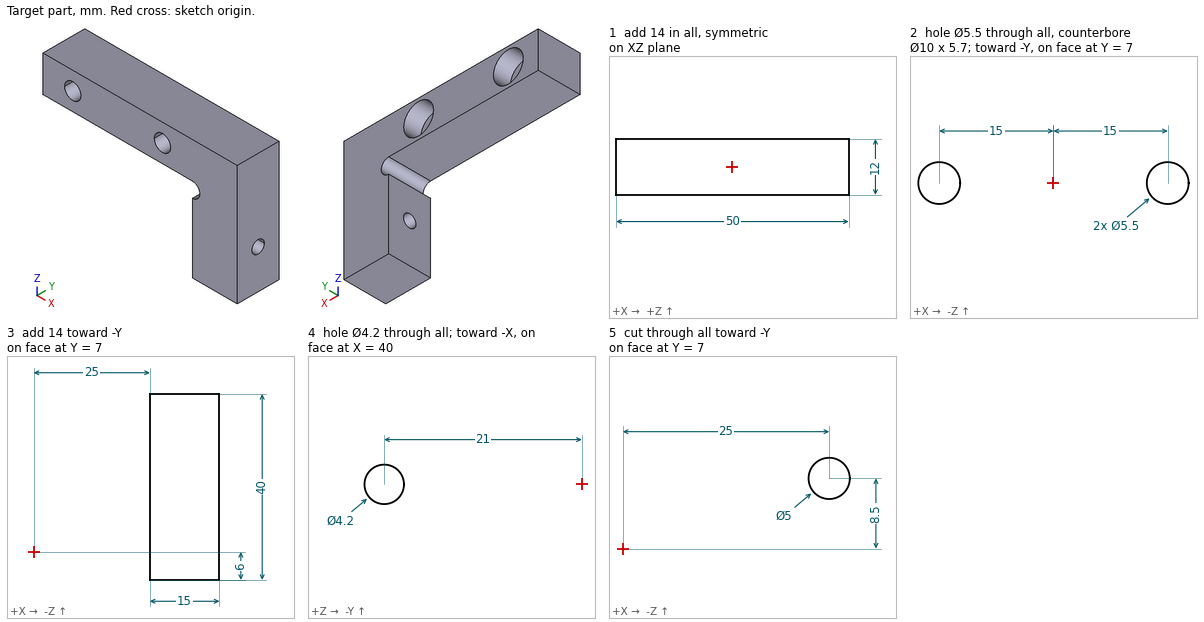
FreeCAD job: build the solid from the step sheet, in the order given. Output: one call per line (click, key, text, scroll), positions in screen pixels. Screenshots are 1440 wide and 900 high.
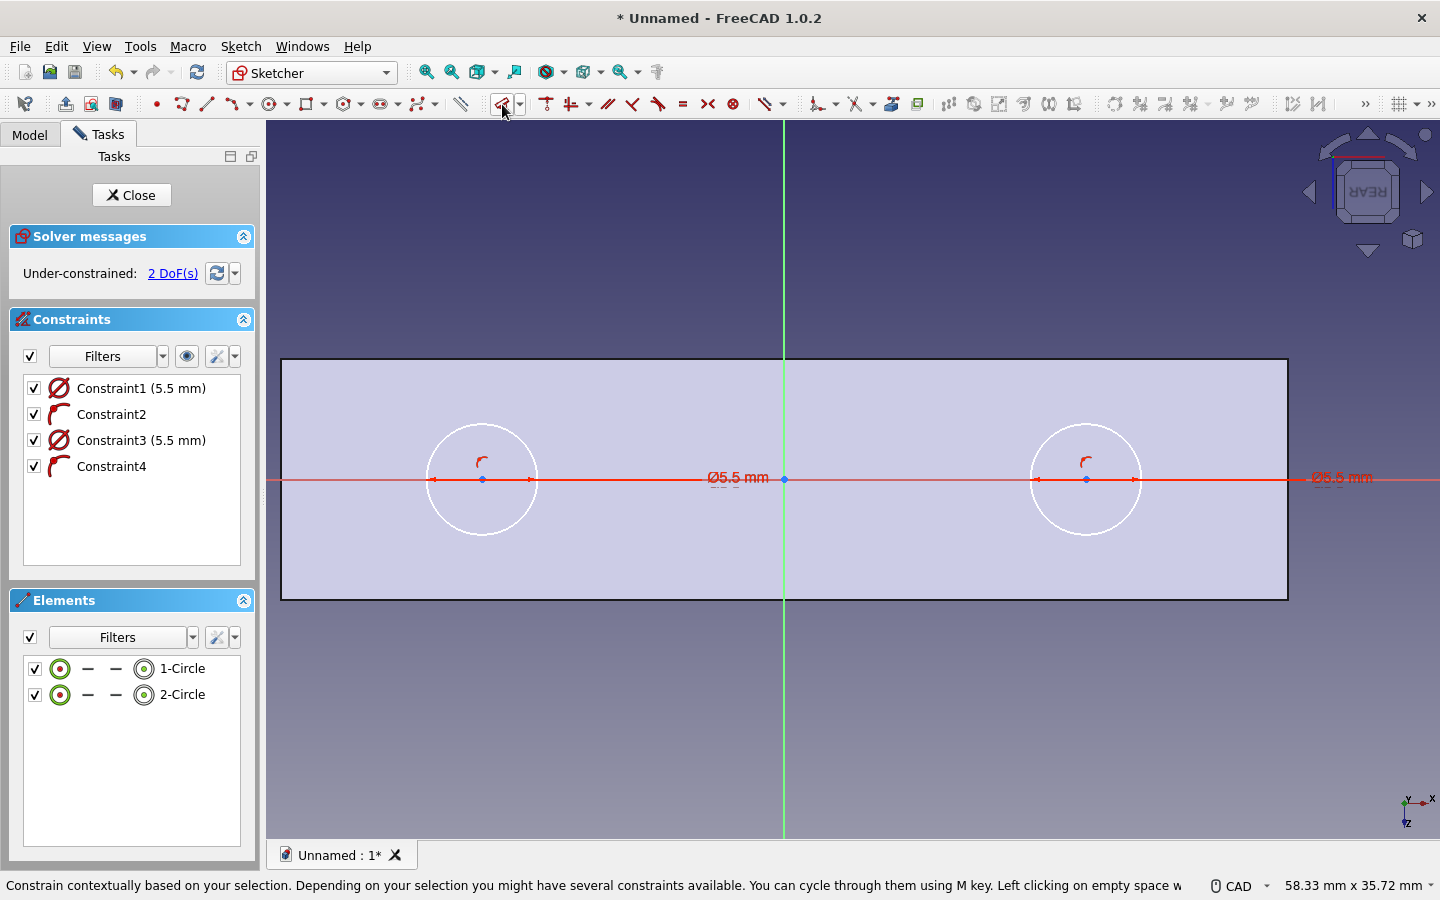
click(1086, 479)
click(935, 513)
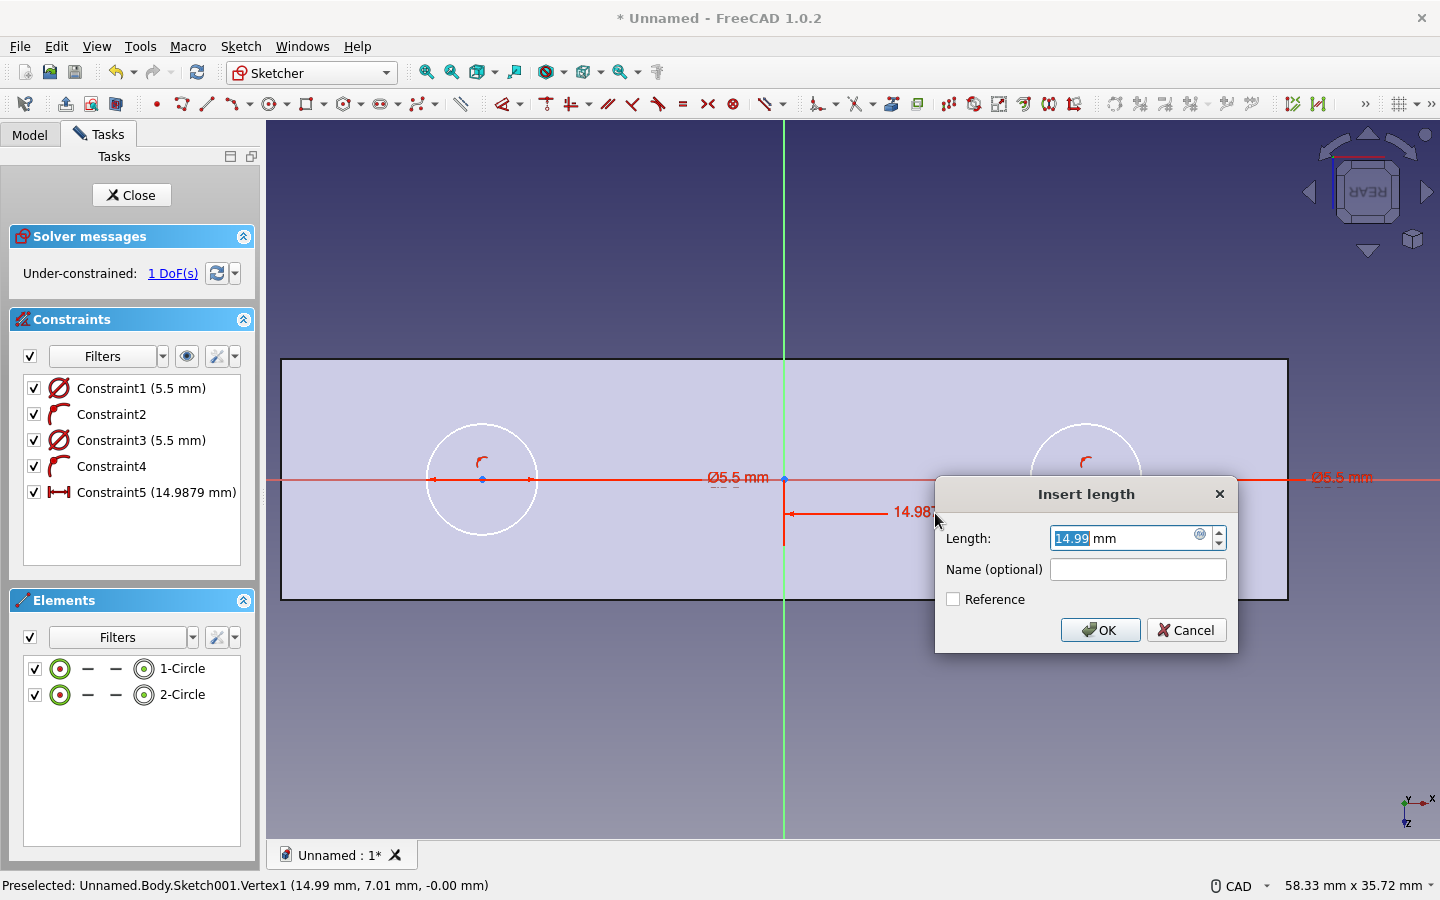
text(15)
key(Return)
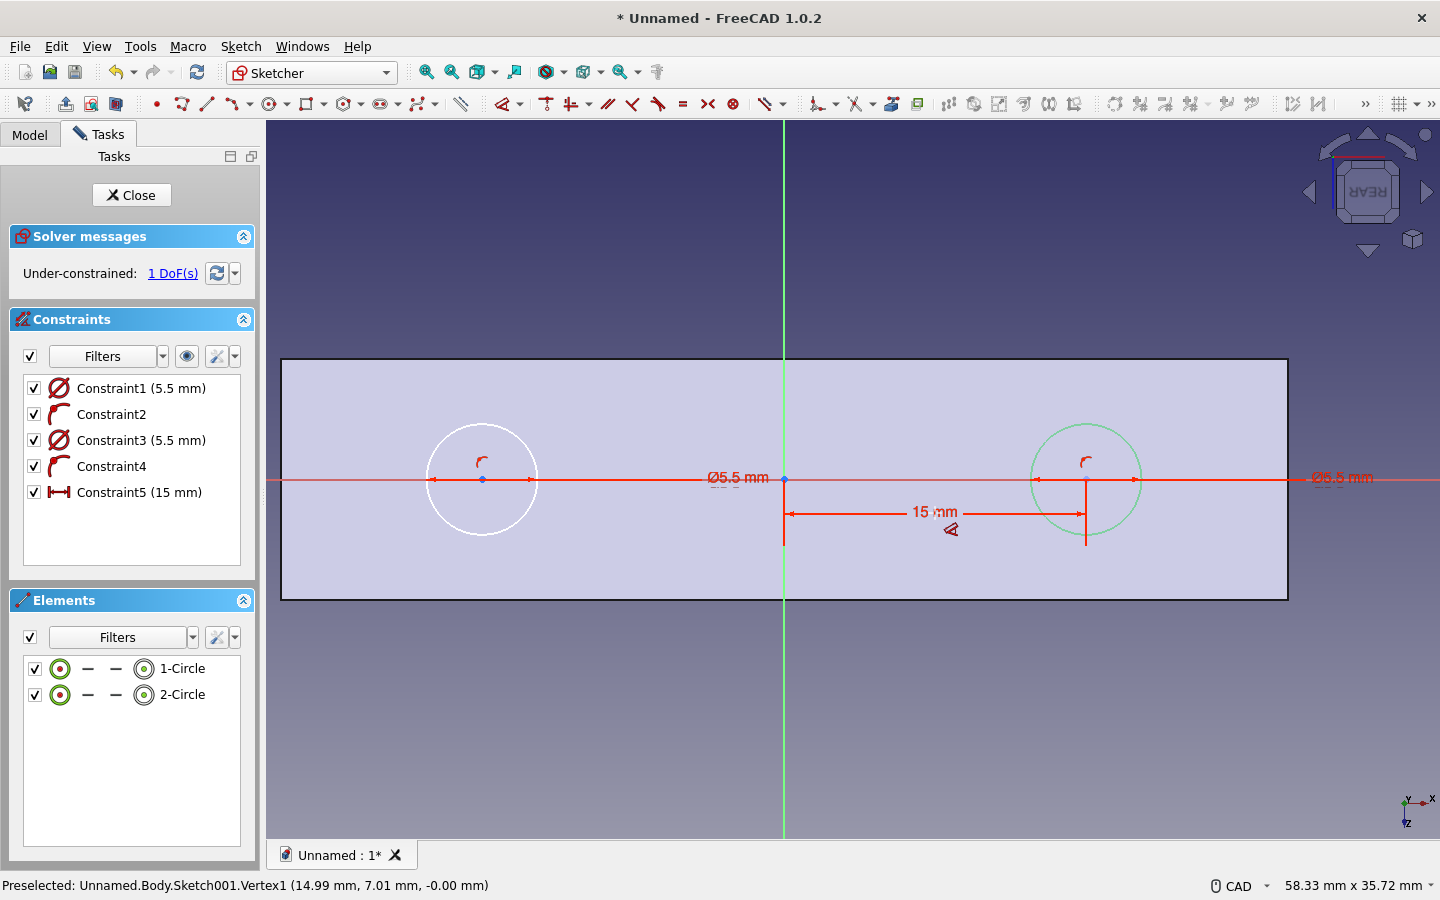
click(482, 479)
click(633, 513)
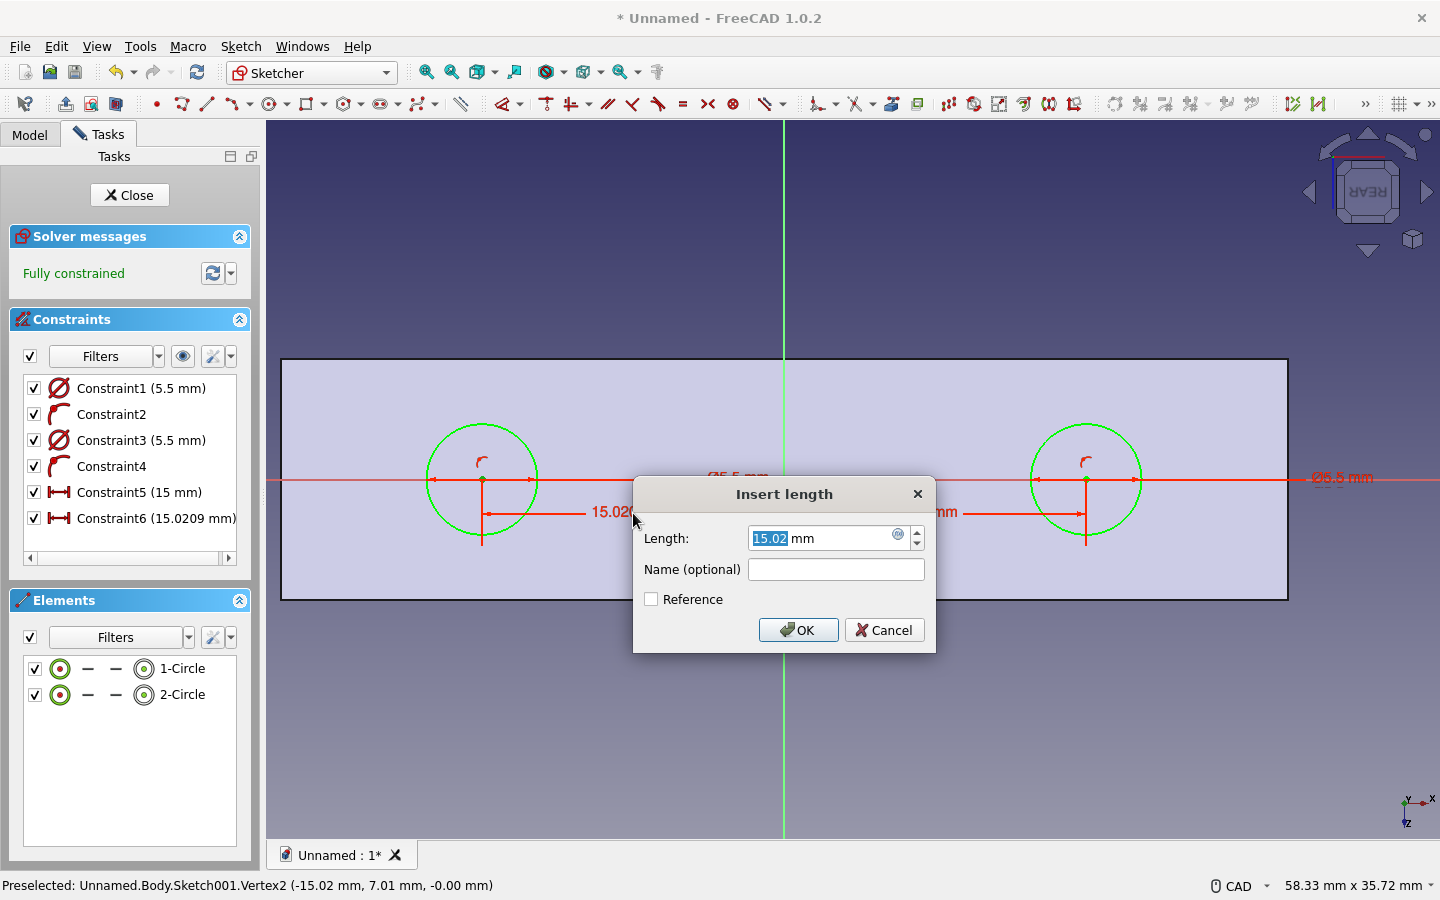
text(15)
key(Return)
key(Escape)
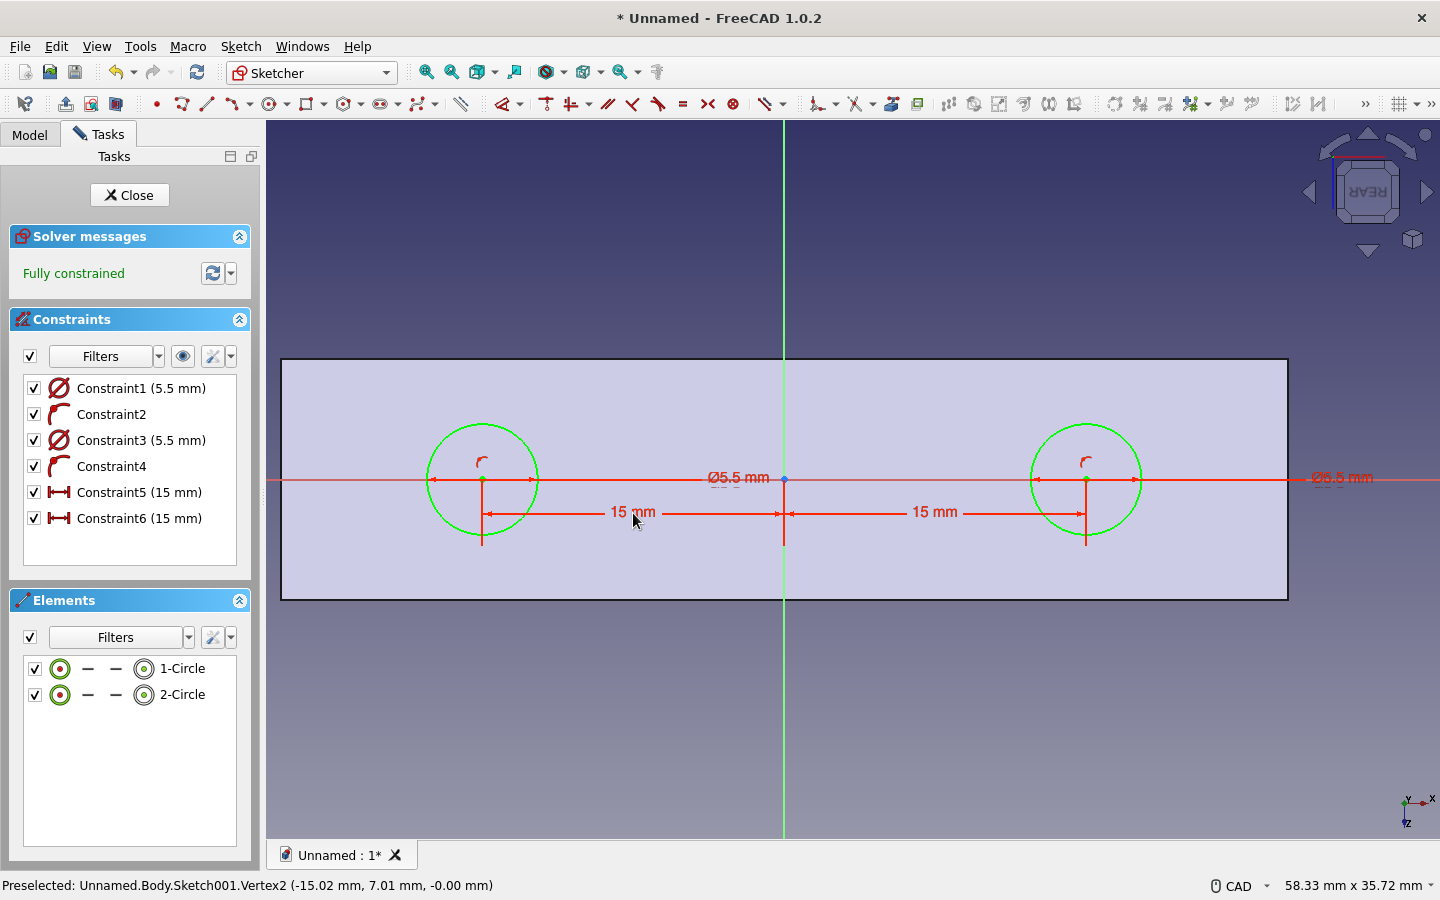
click(130, 195)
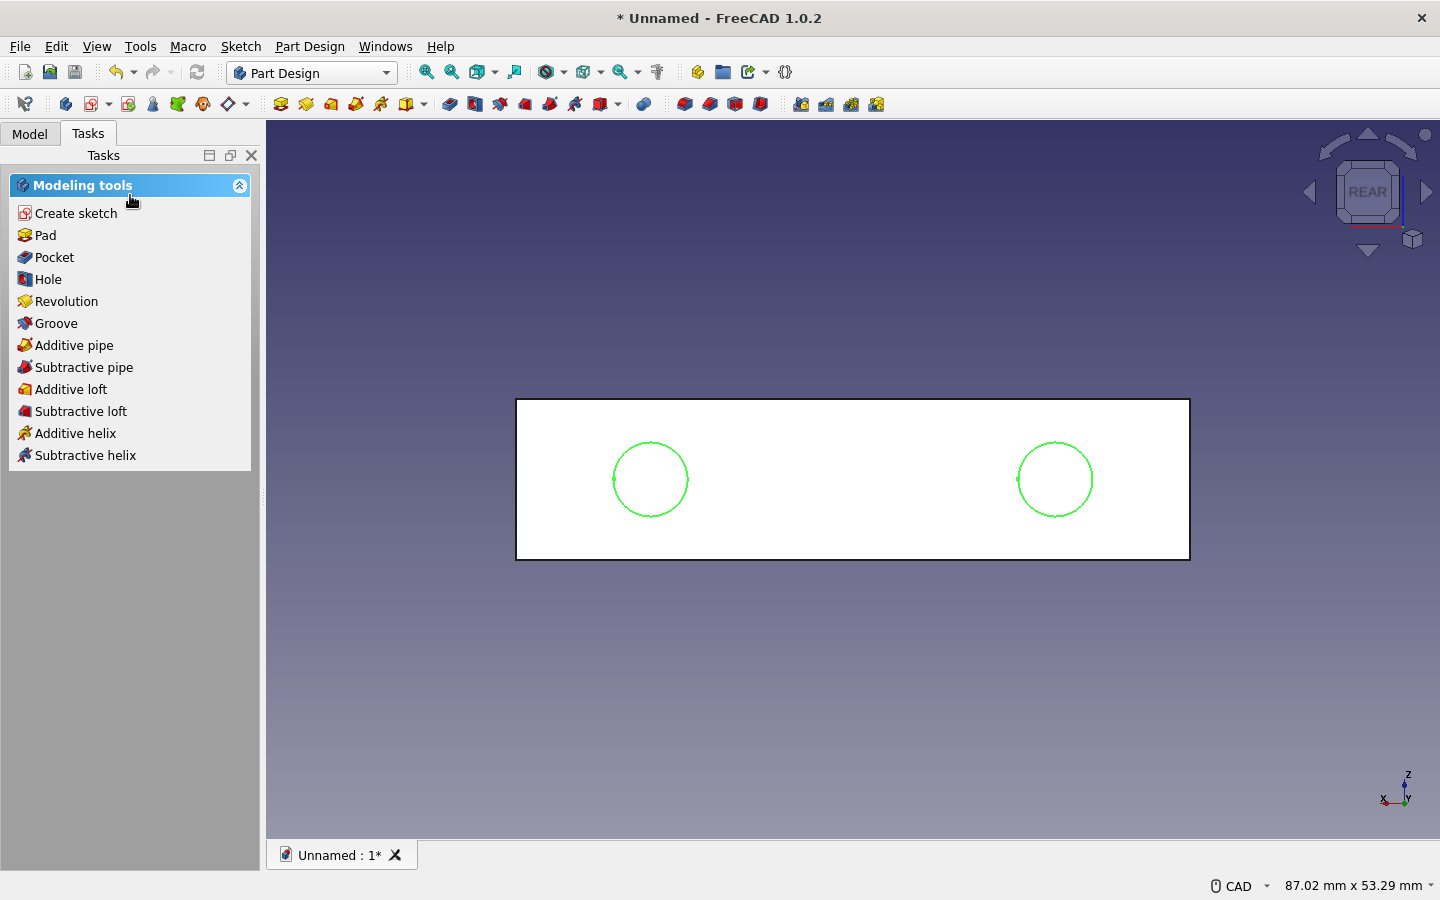
click(475, 104)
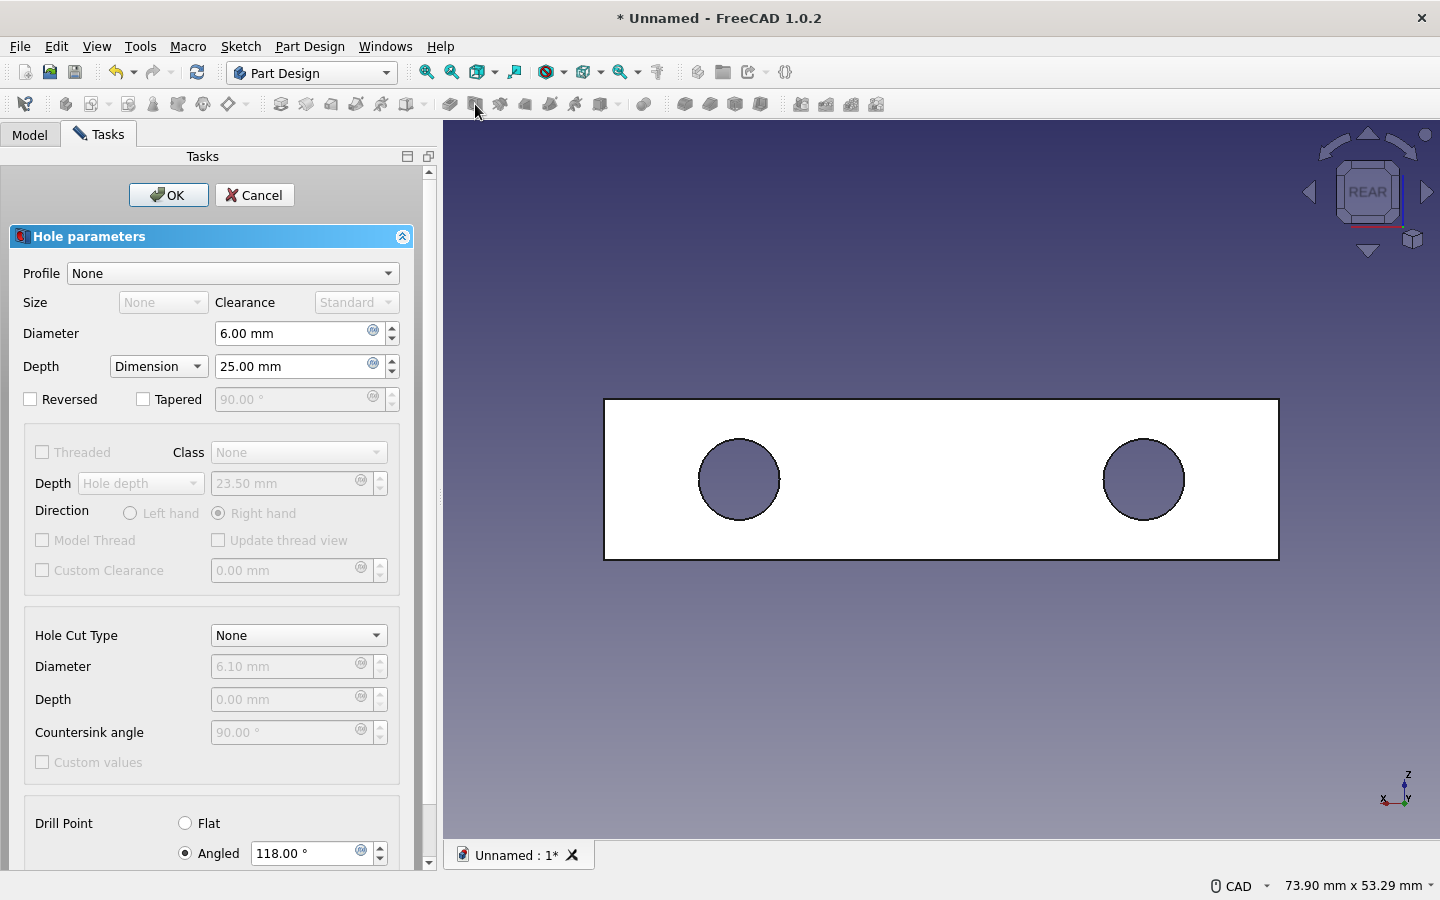
triple_click(300, 334)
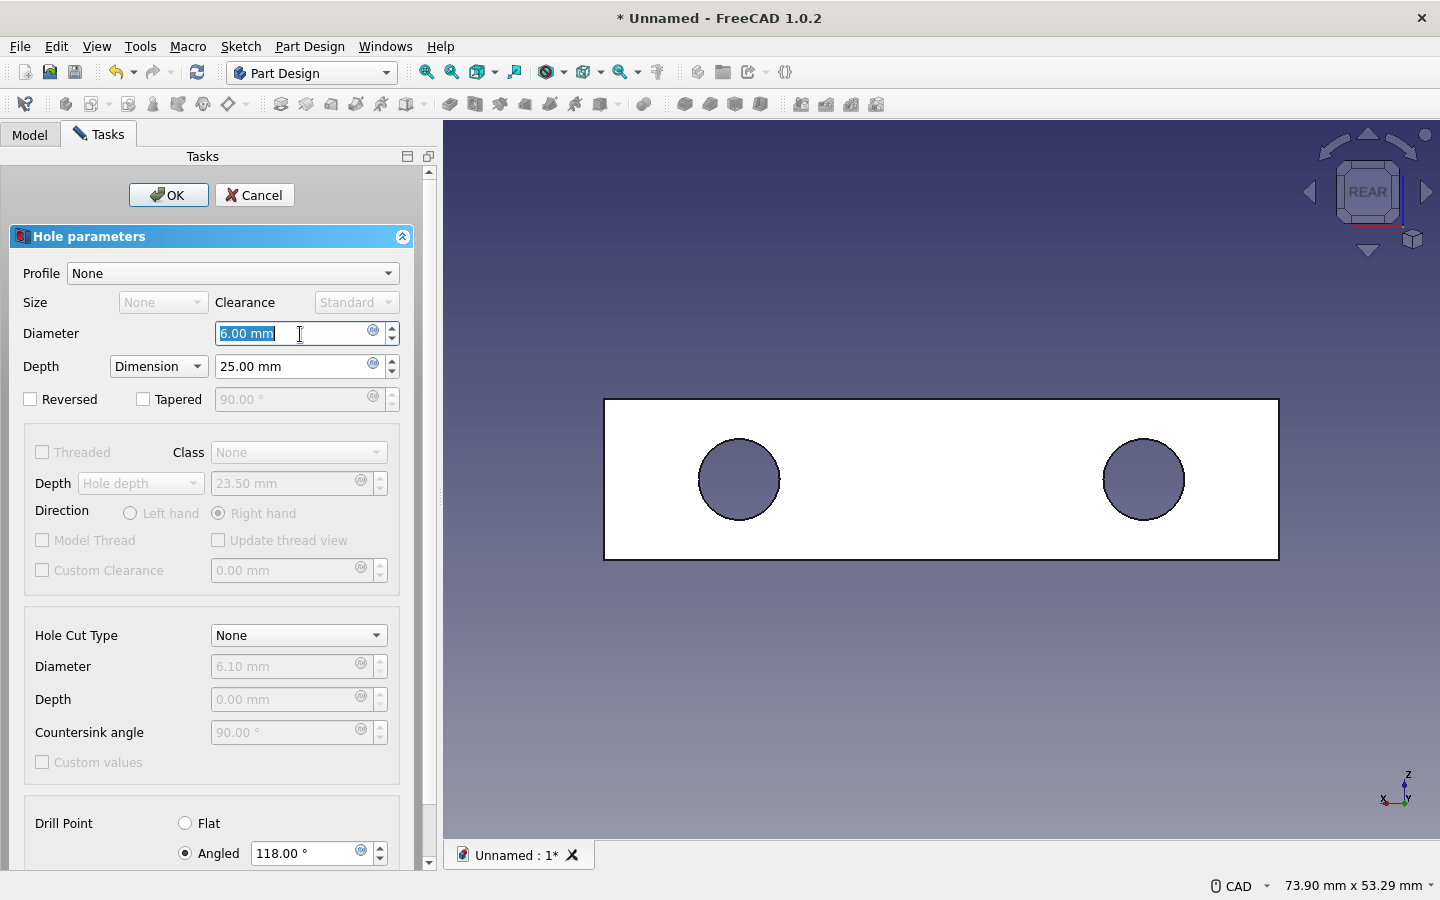
text(5.5)
key(Tab)